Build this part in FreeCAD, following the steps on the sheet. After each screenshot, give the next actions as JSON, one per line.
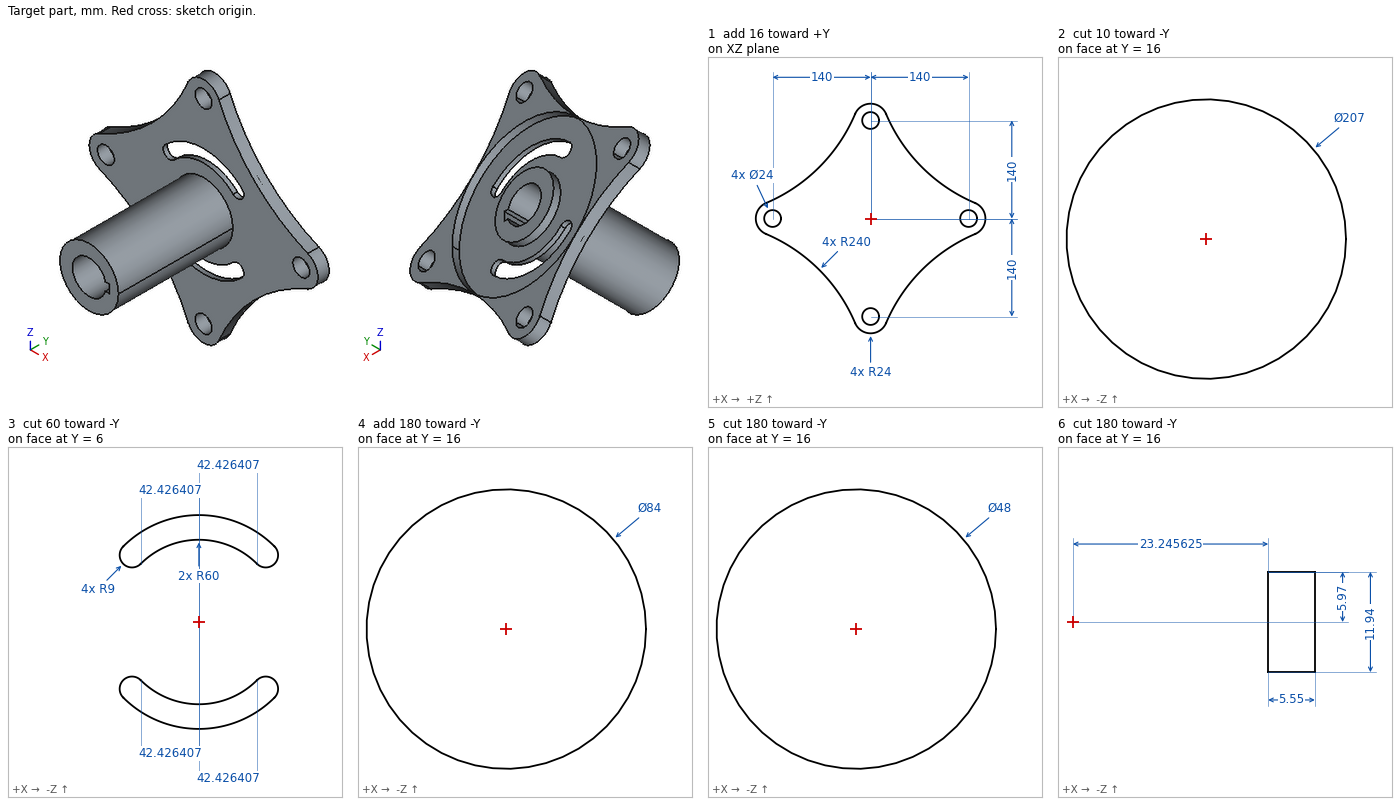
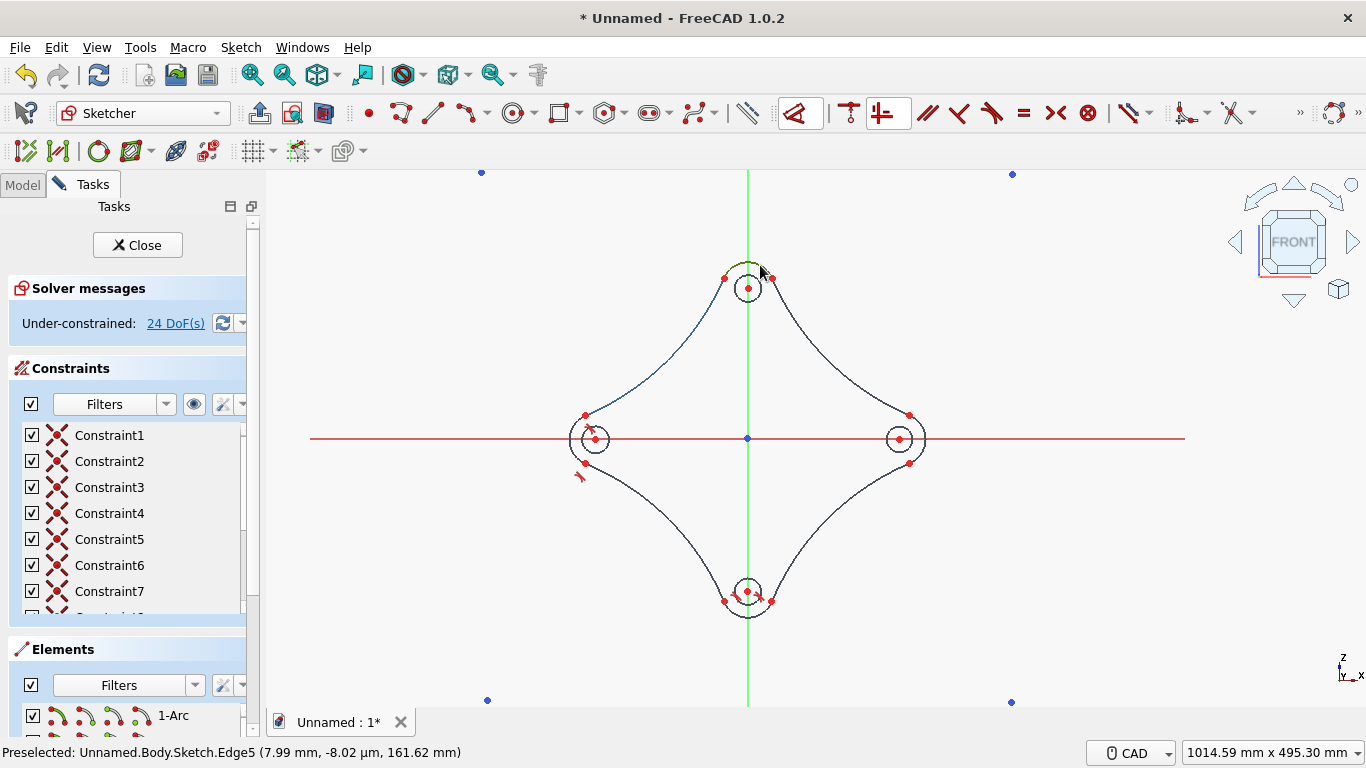
{"action": "left_click", "coordinate": [992, 114]}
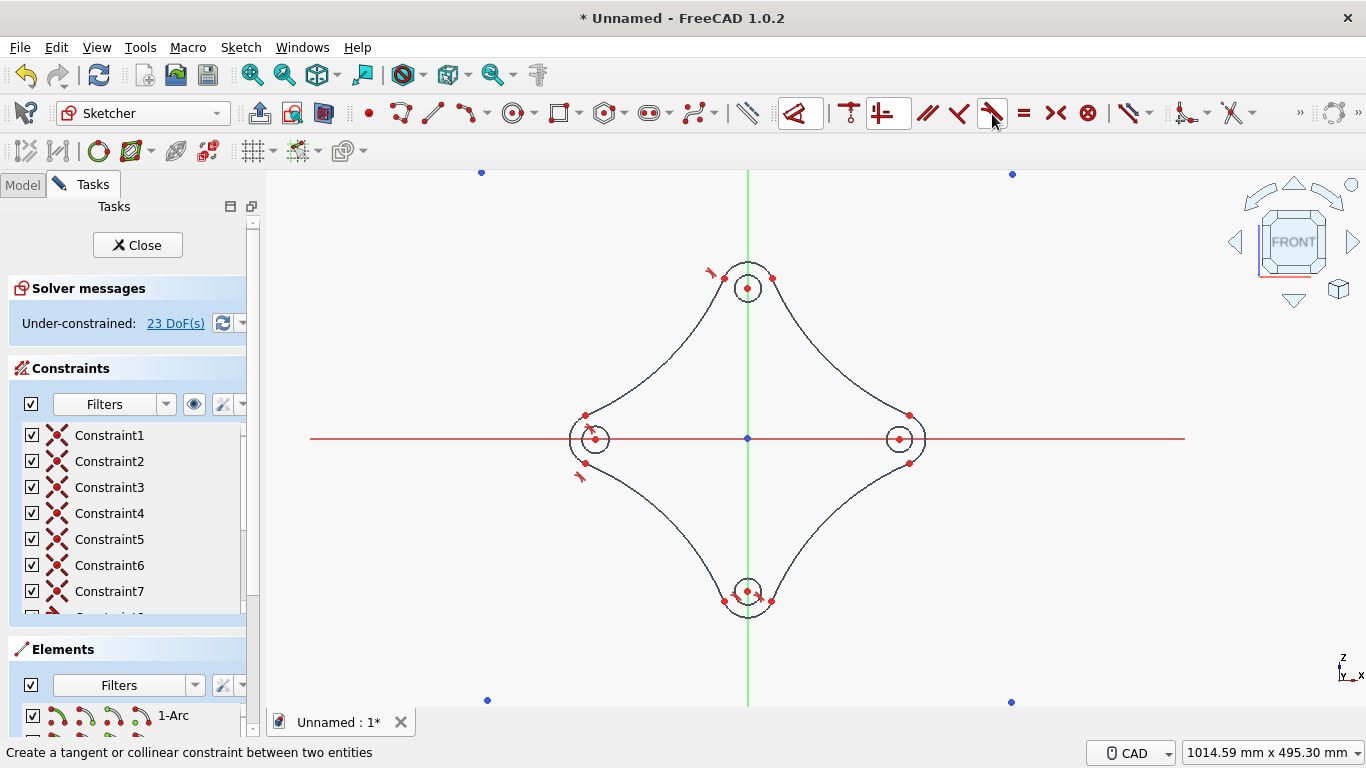
{"action": "left_click", "coordinate": [760, 265]}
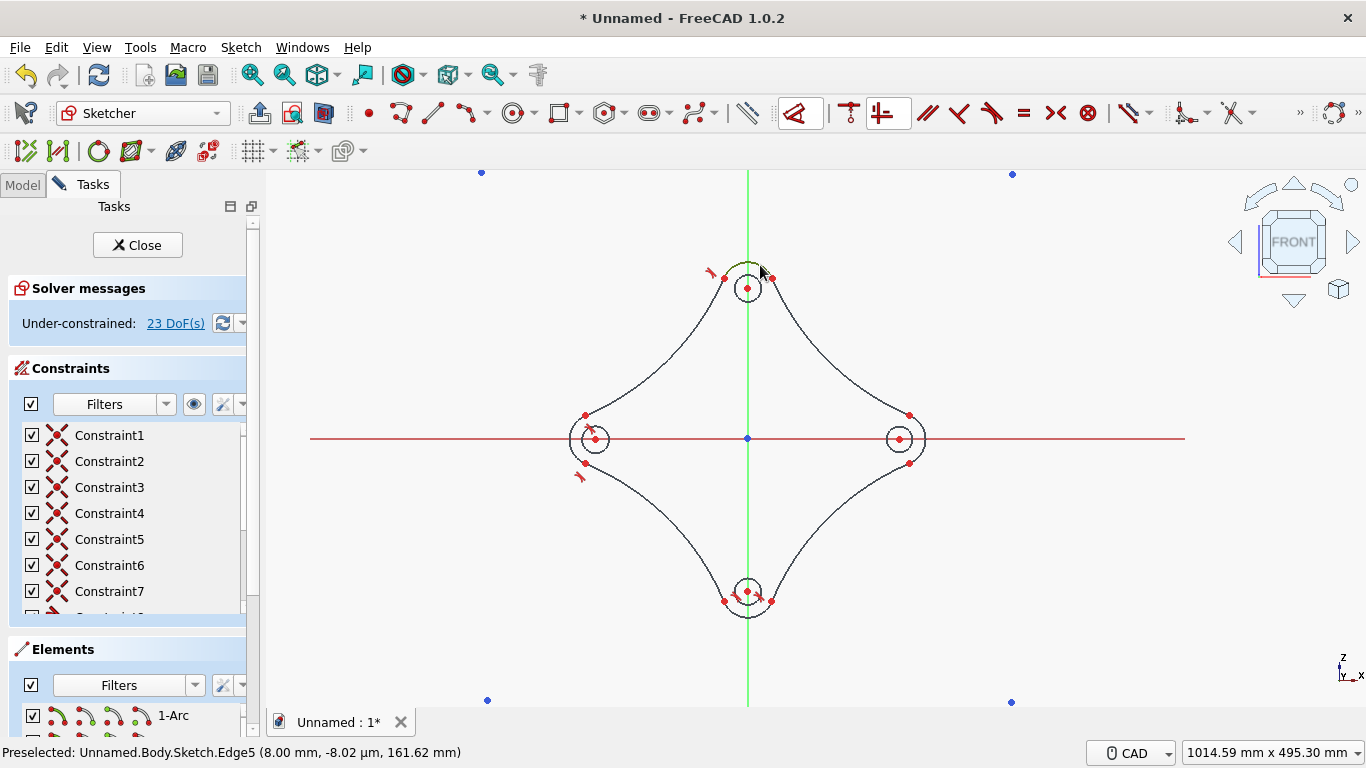
{"action": "left_click", "coordinate": [802, 330]}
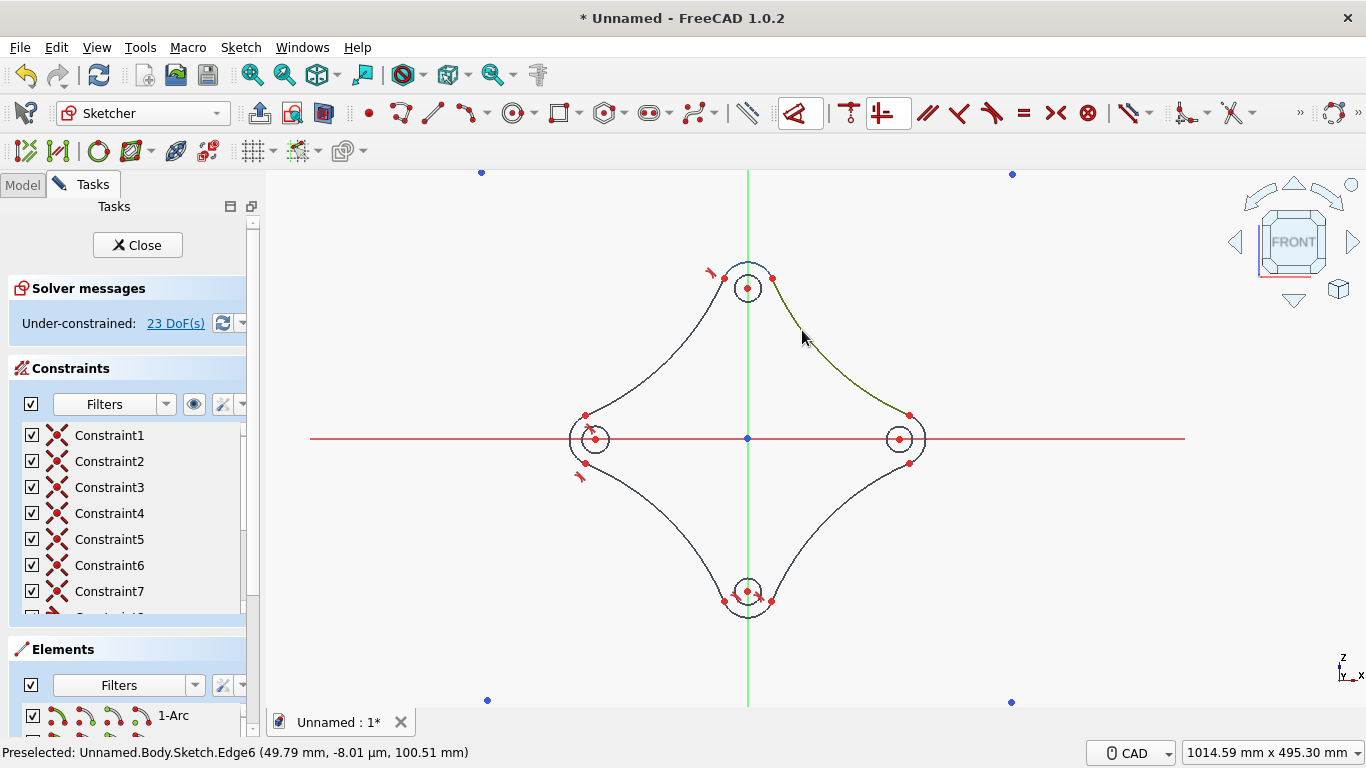
{"action": "left_click", "coordinate": [992, 114]}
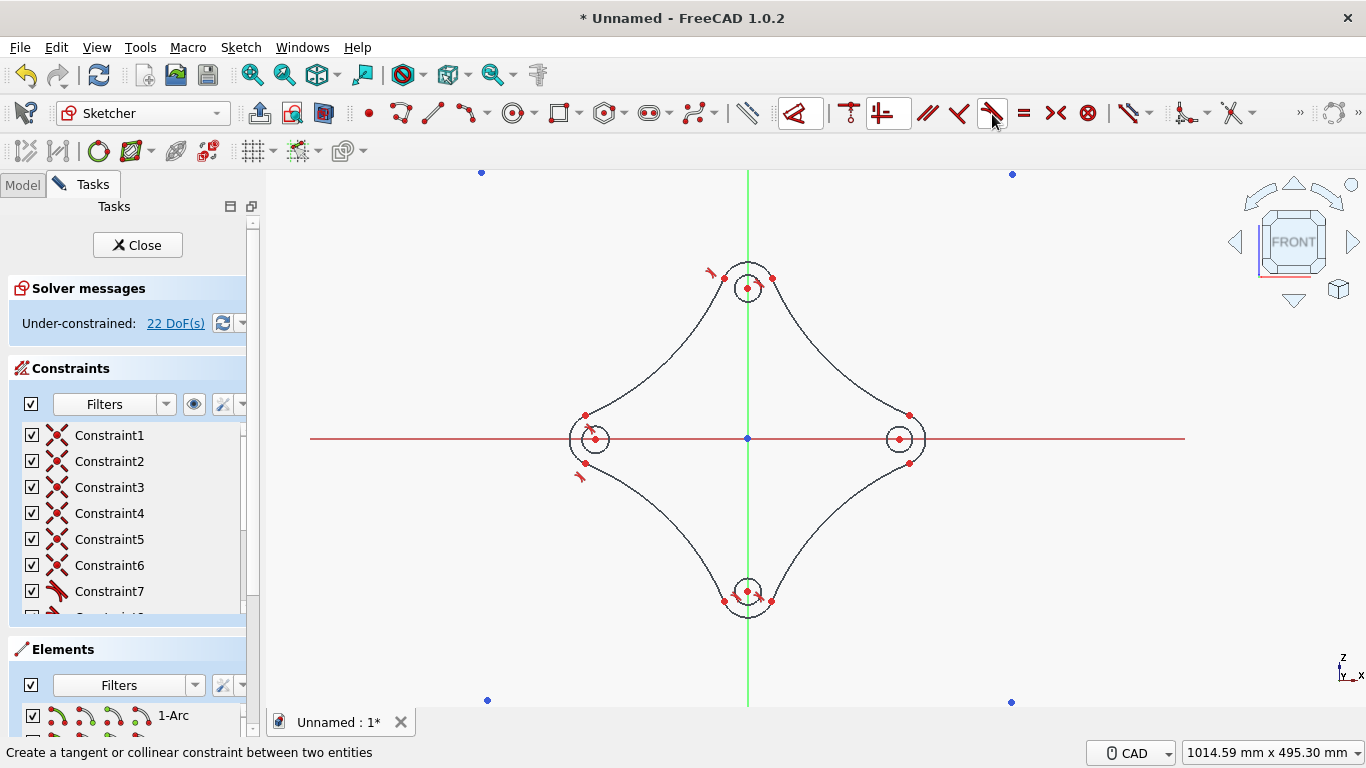
{"action": "left_click", "coordinate": [802, 330]}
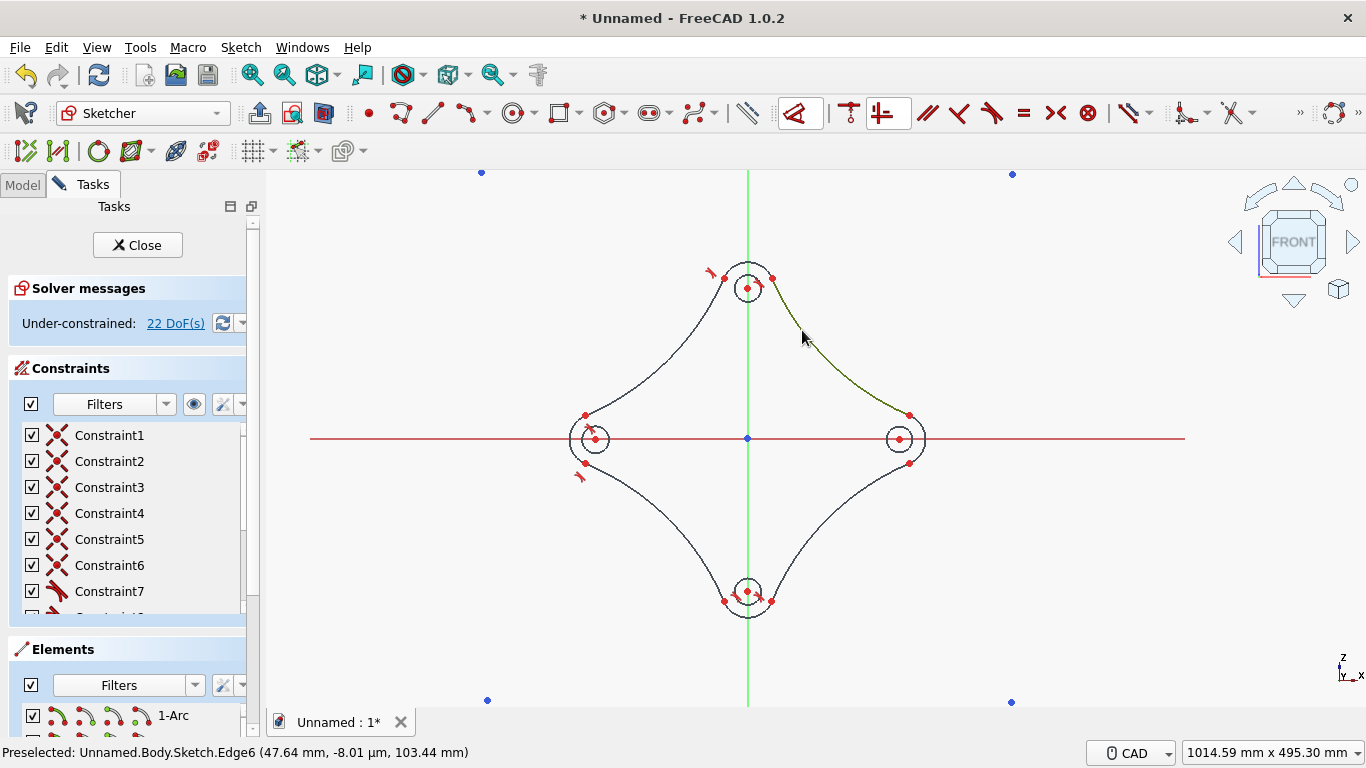
{"action": "left_click", "coordinate": [923, 451]}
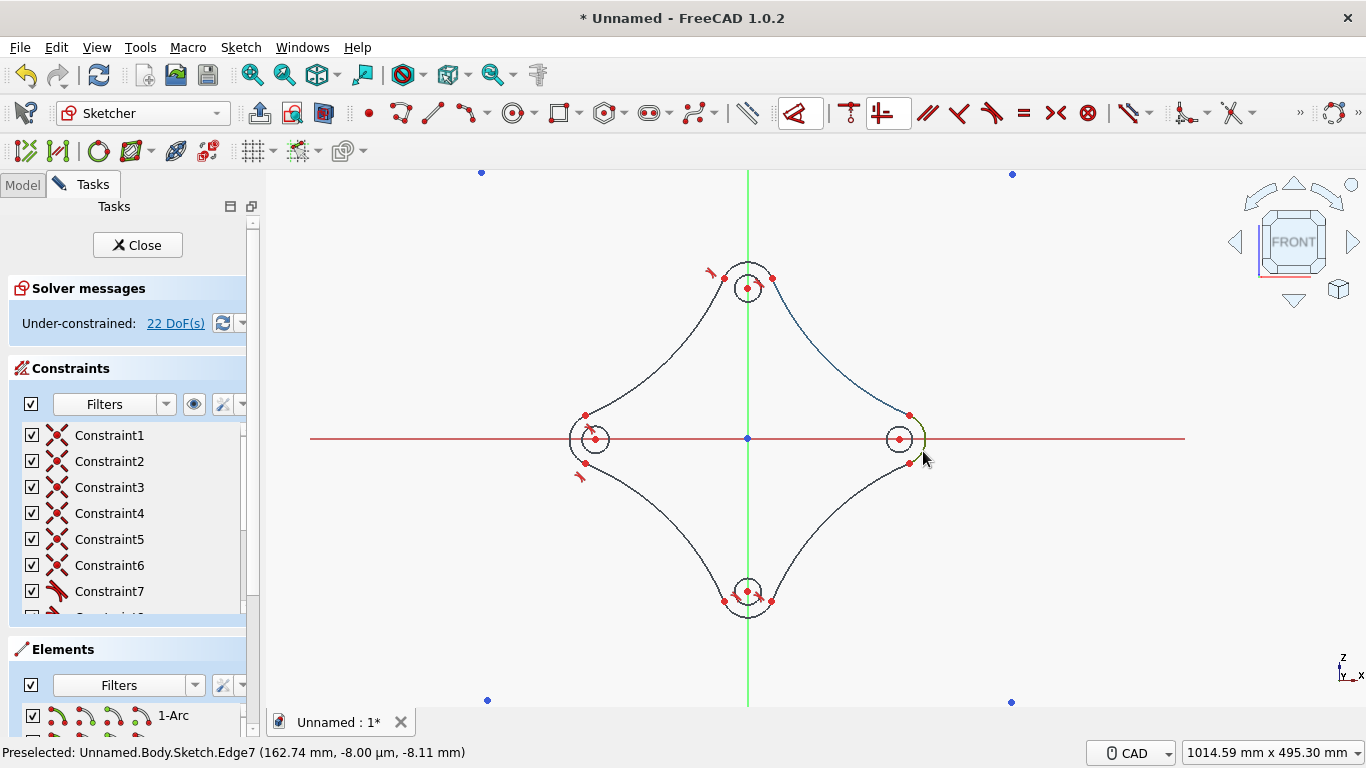
{"action": "left_click", "coordinate": [992, 114]}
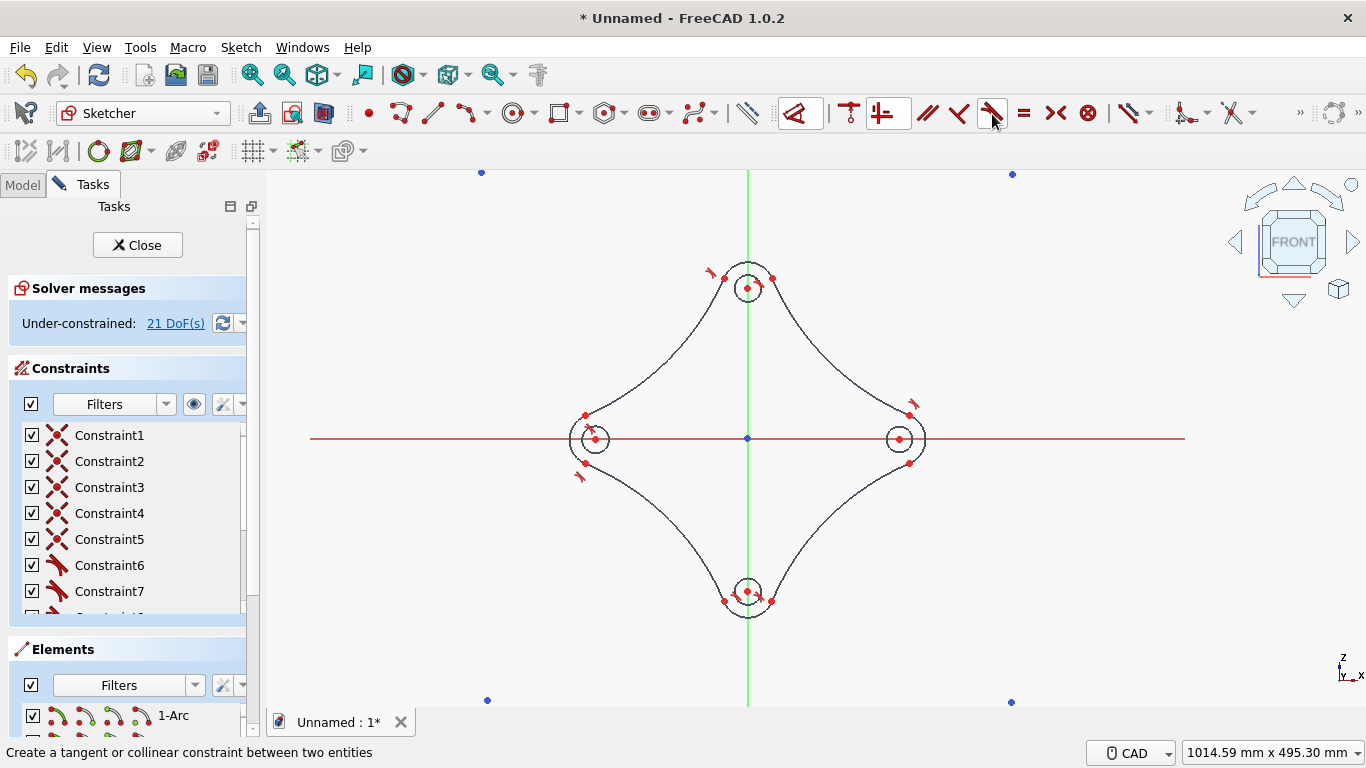
{"action": "left_click", "coordinate": [923, 451]}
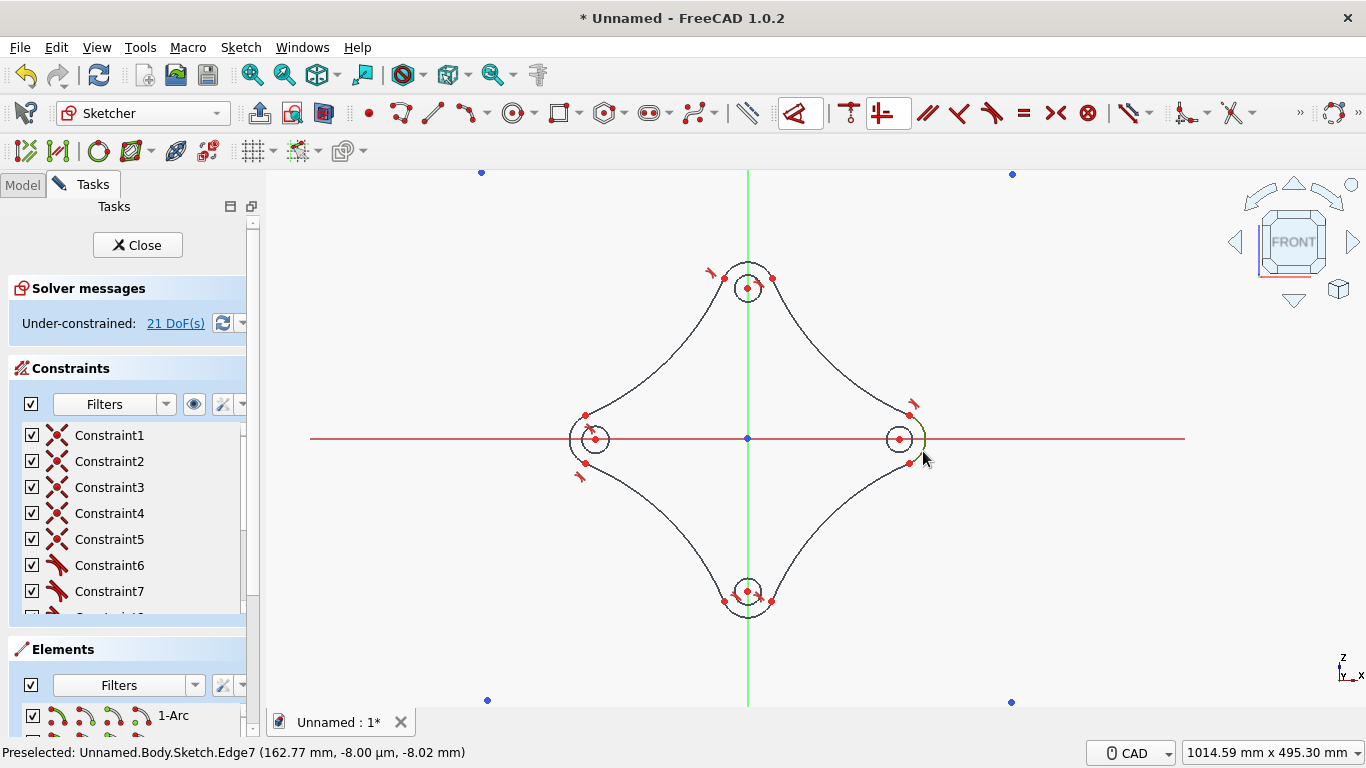
{"action": "left_click", "coordinate": [858, 493]}